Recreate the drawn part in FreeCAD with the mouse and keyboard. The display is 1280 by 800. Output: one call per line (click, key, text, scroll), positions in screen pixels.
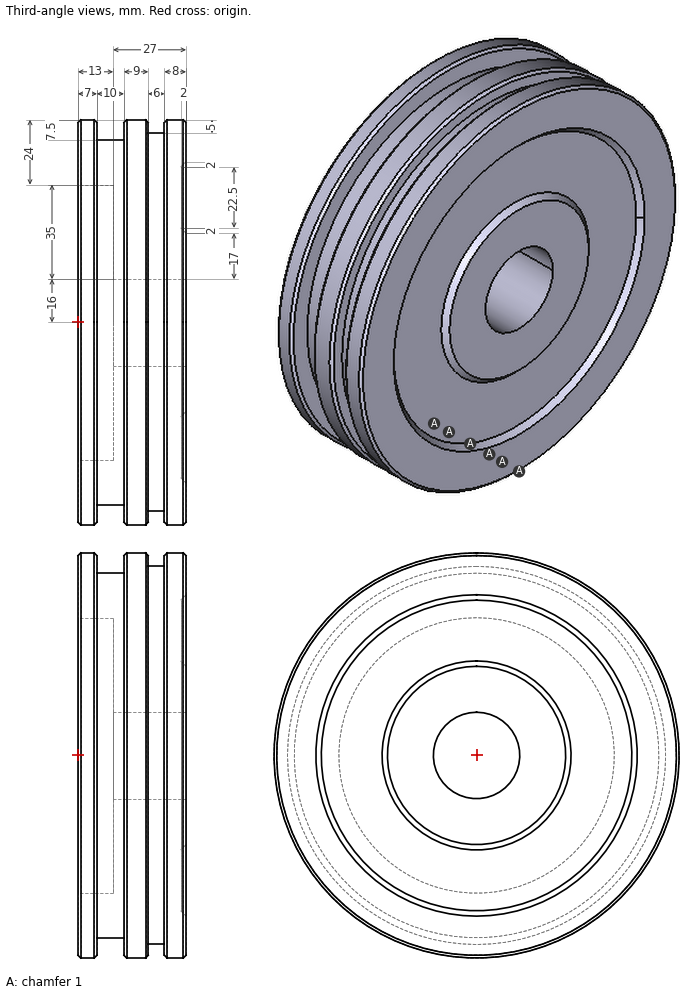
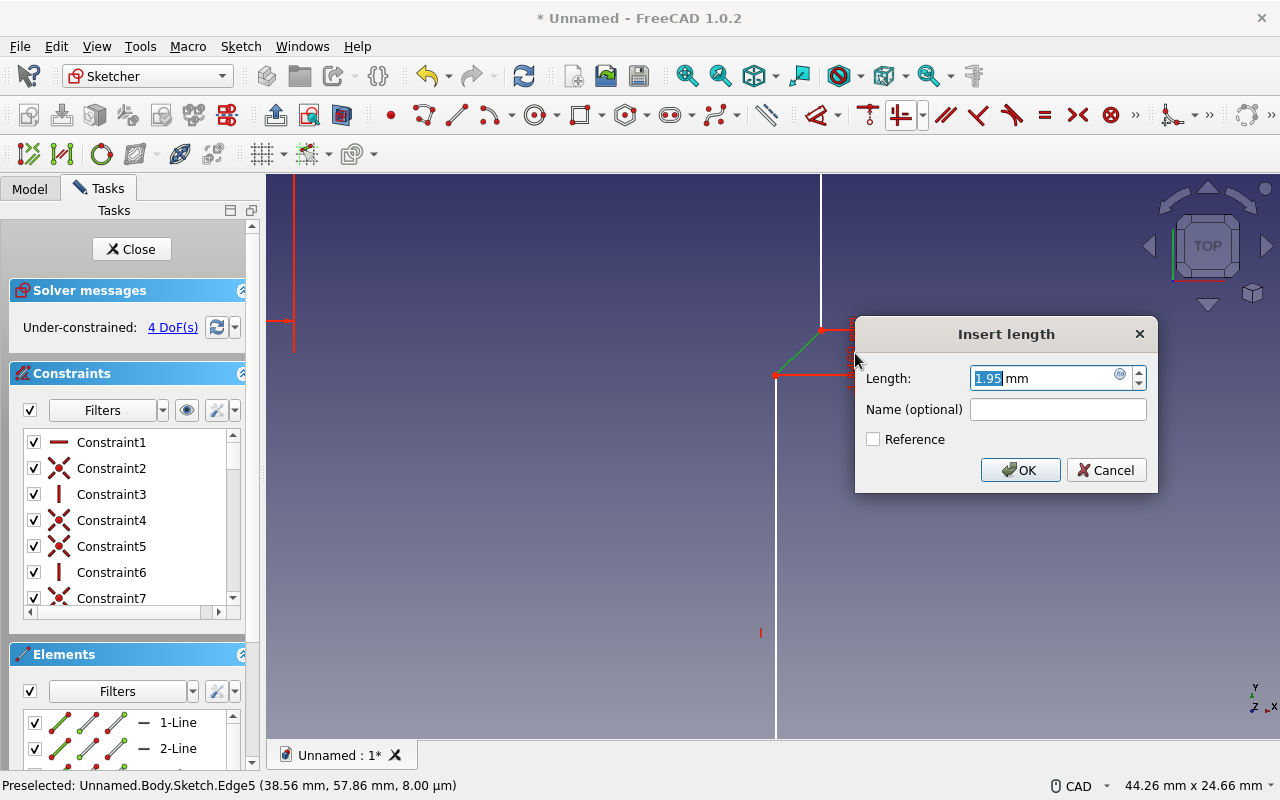
text(2)
key(Return)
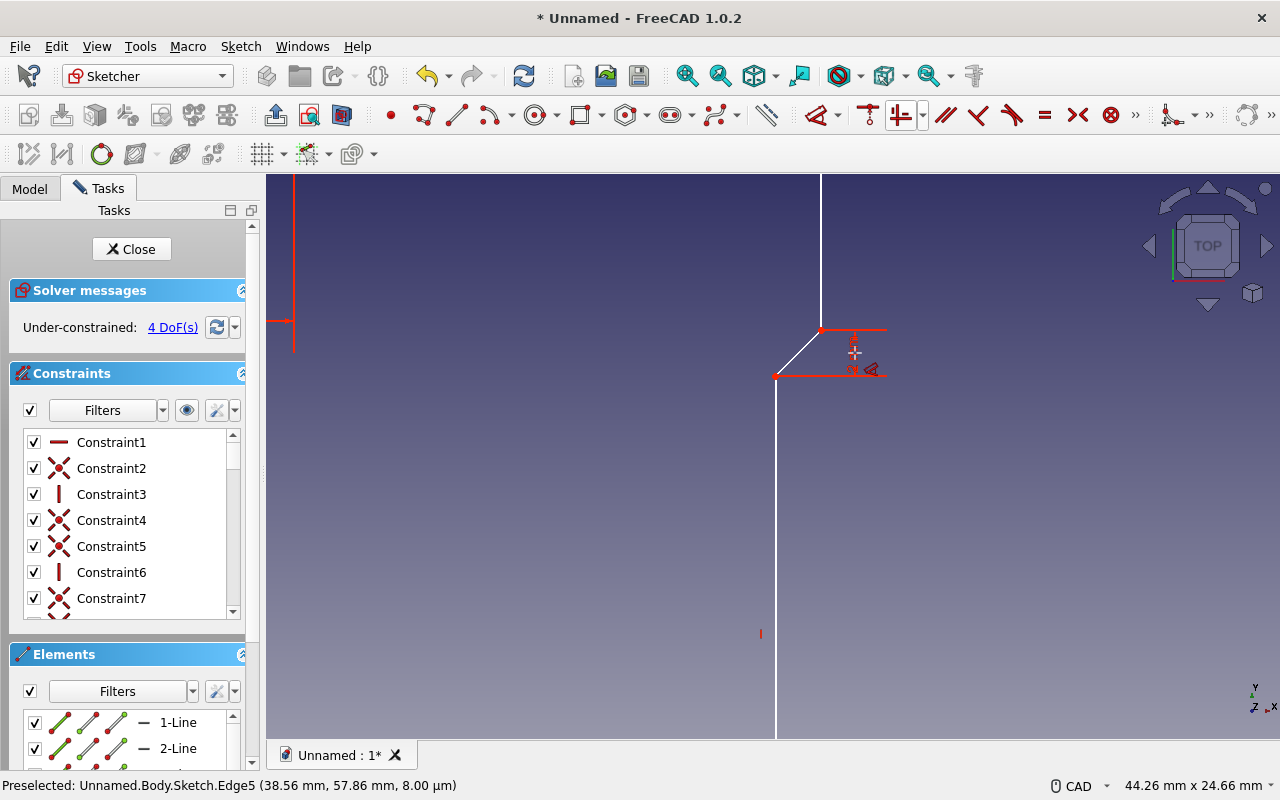
scroll(791, 362, down, 8)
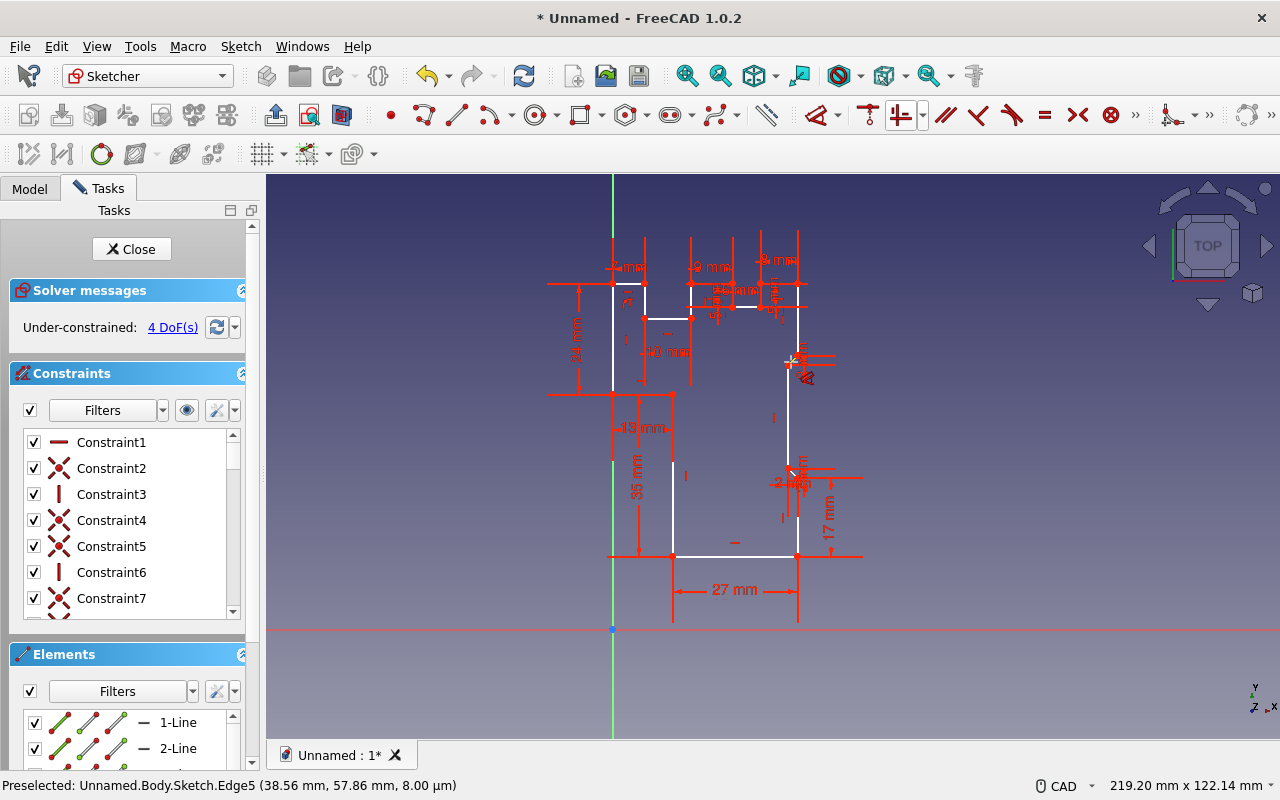
scroll(691, 294, up, 2)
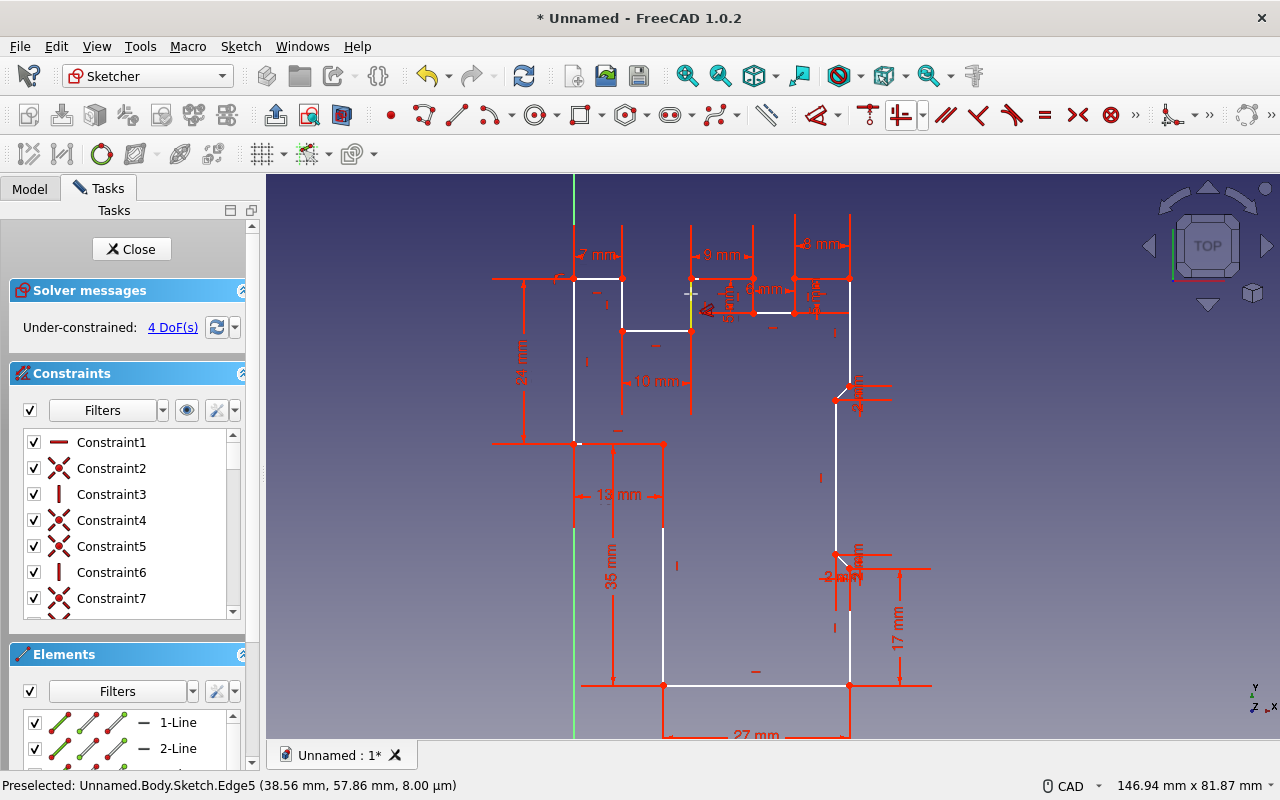
click(691, 295)
click(657, 305)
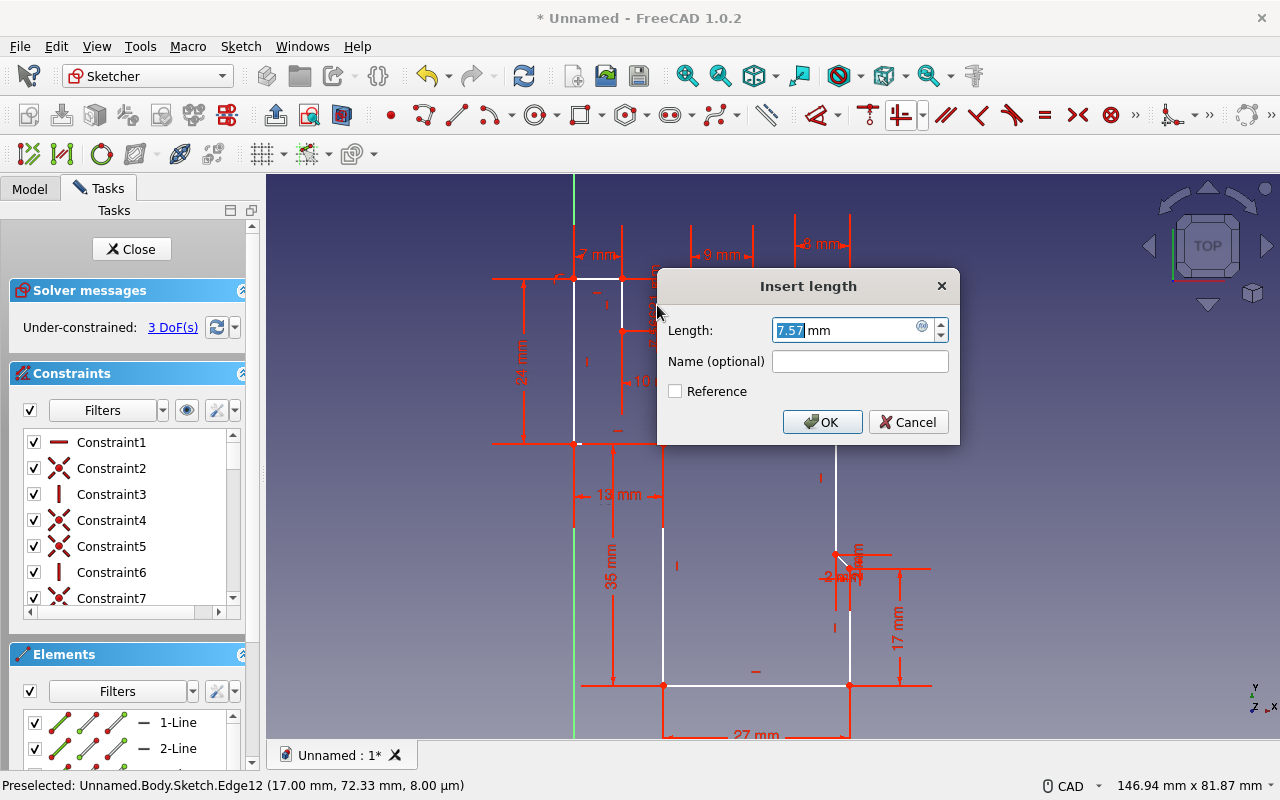
text(7.5)
key(Return)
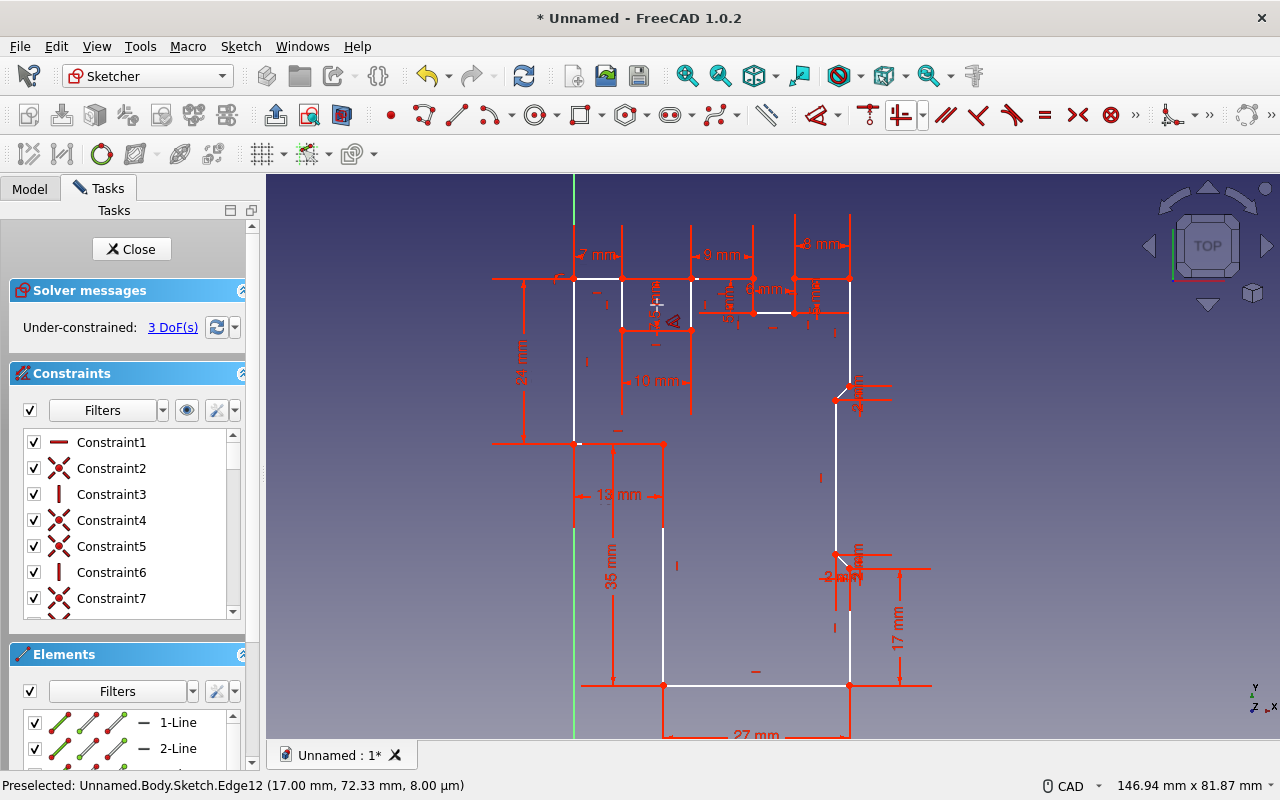
click(622, 315)
click(540, 305)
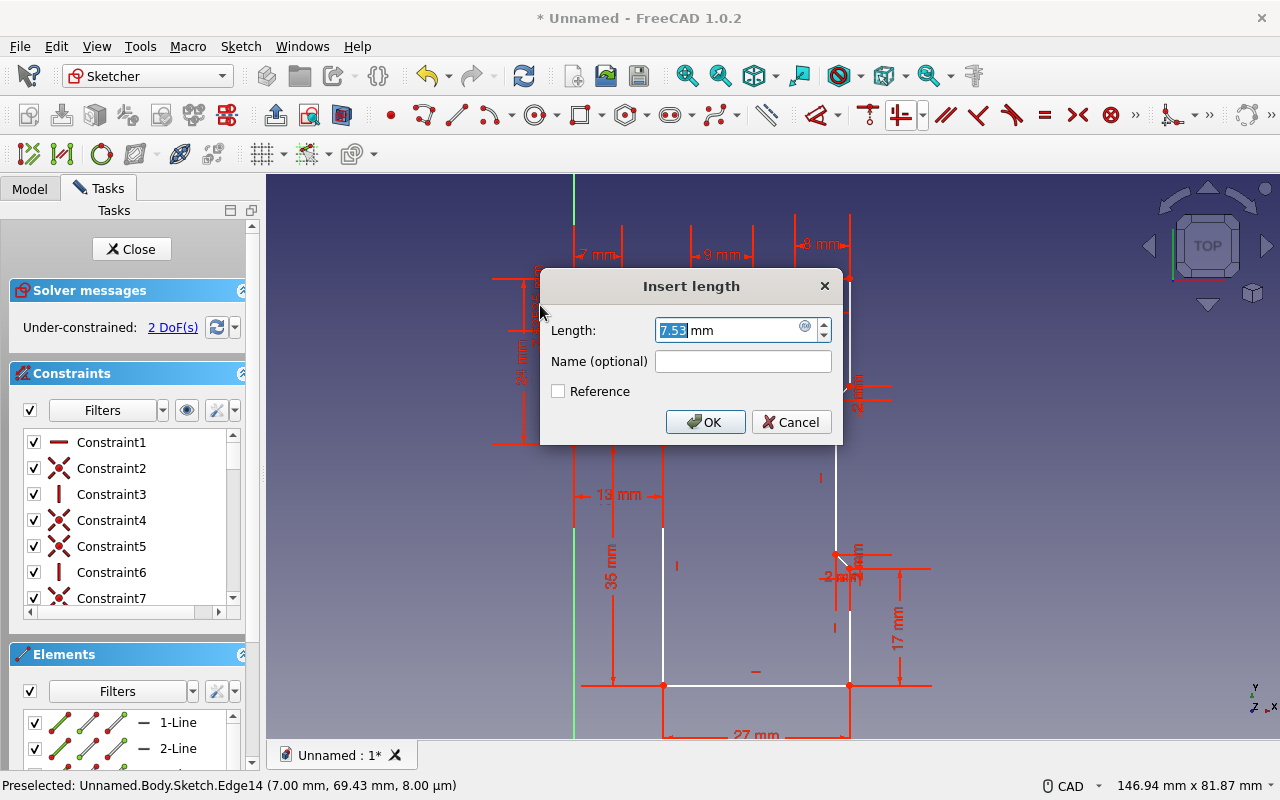
text(7.5)
key(Return)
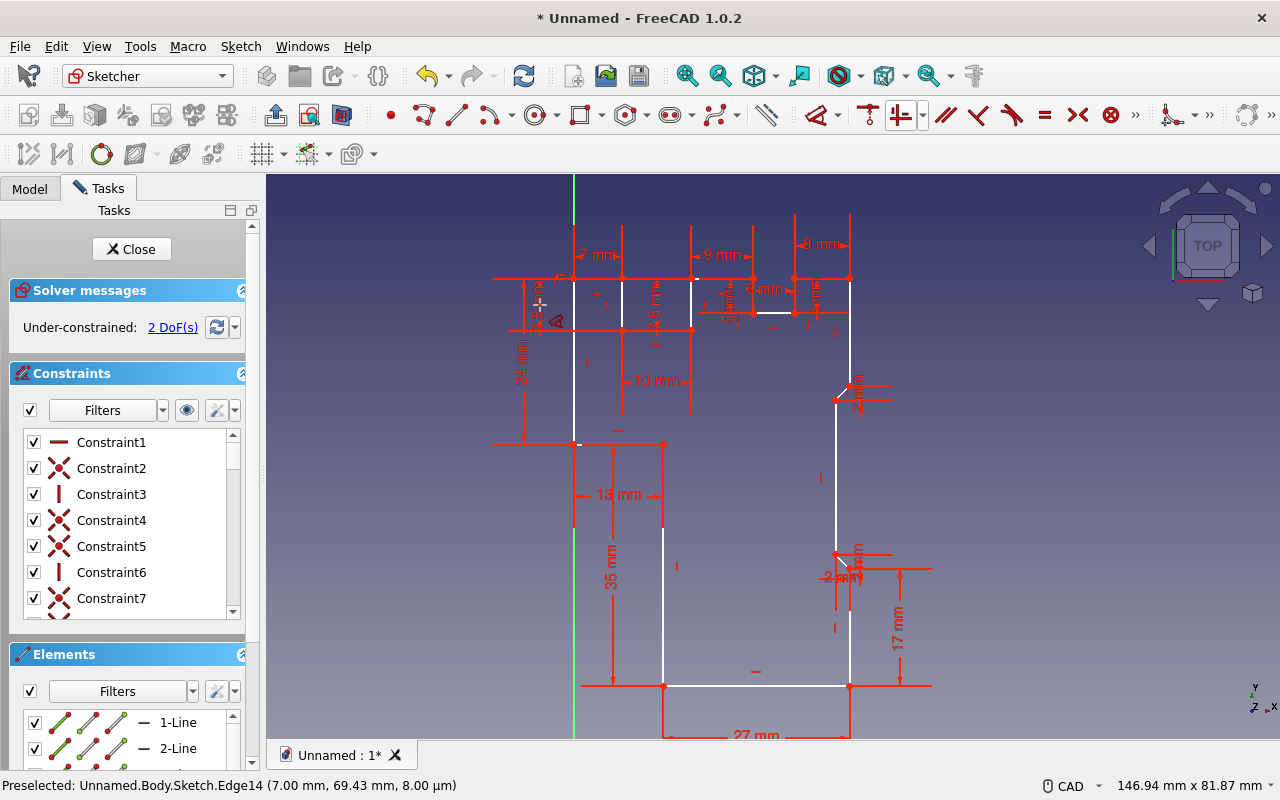
click(663, 686)
click(540, 699)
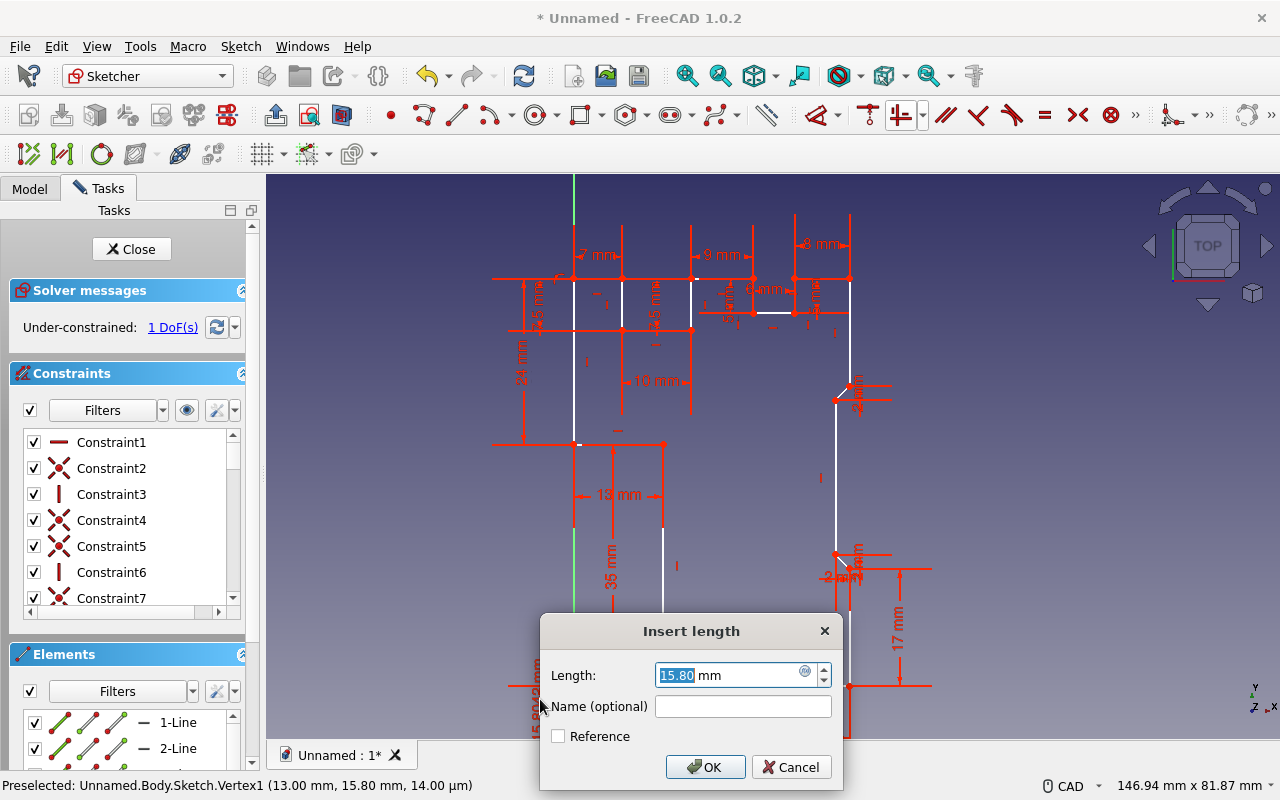
text(16)
key(Return)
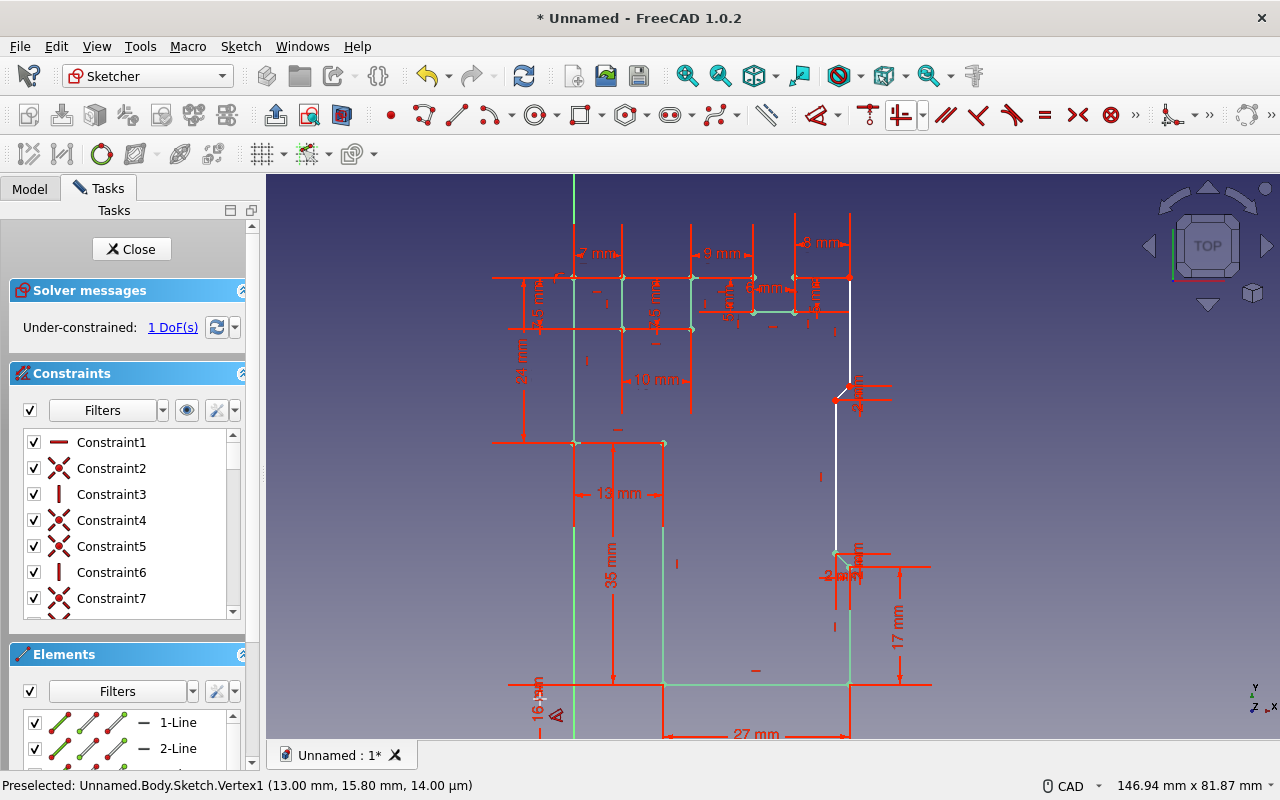
click(836, 508)
click(870, 477)